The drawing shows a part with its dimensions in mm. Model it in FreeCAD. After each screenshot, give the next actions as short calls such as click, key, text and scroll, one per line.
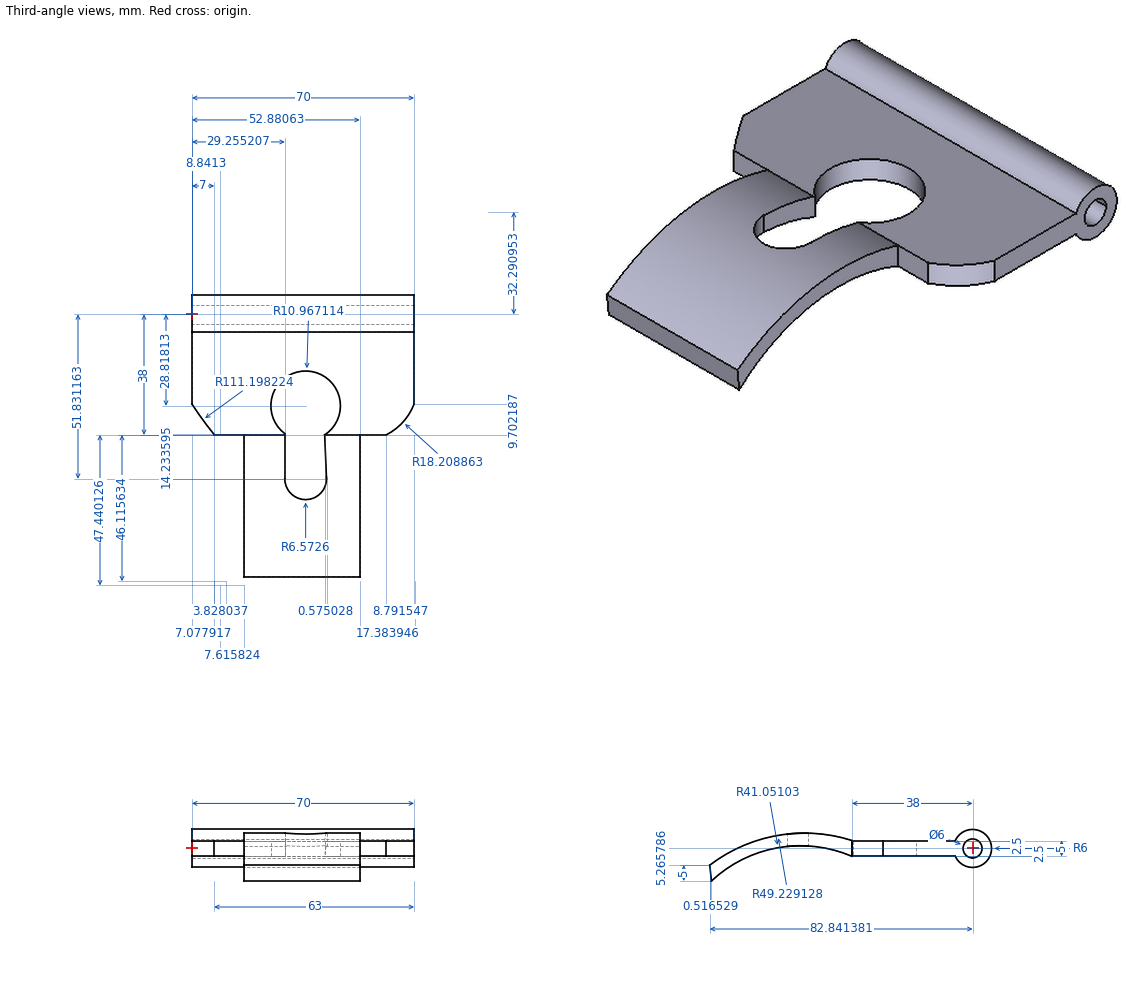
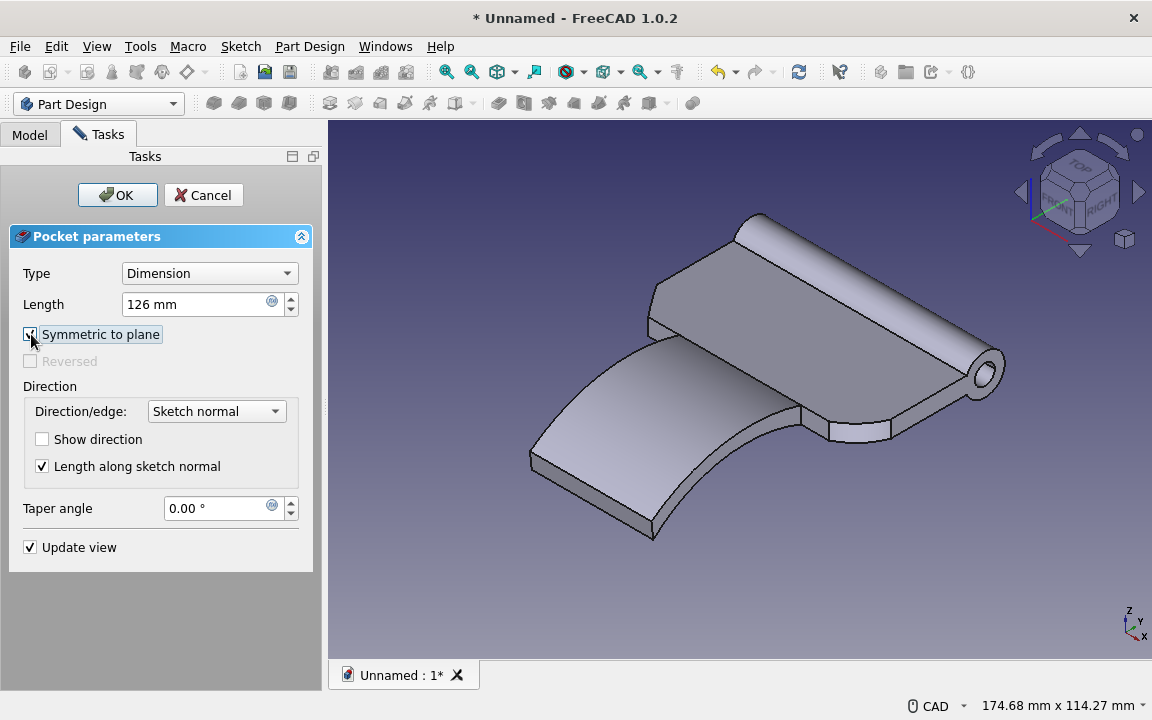
click(118, 195)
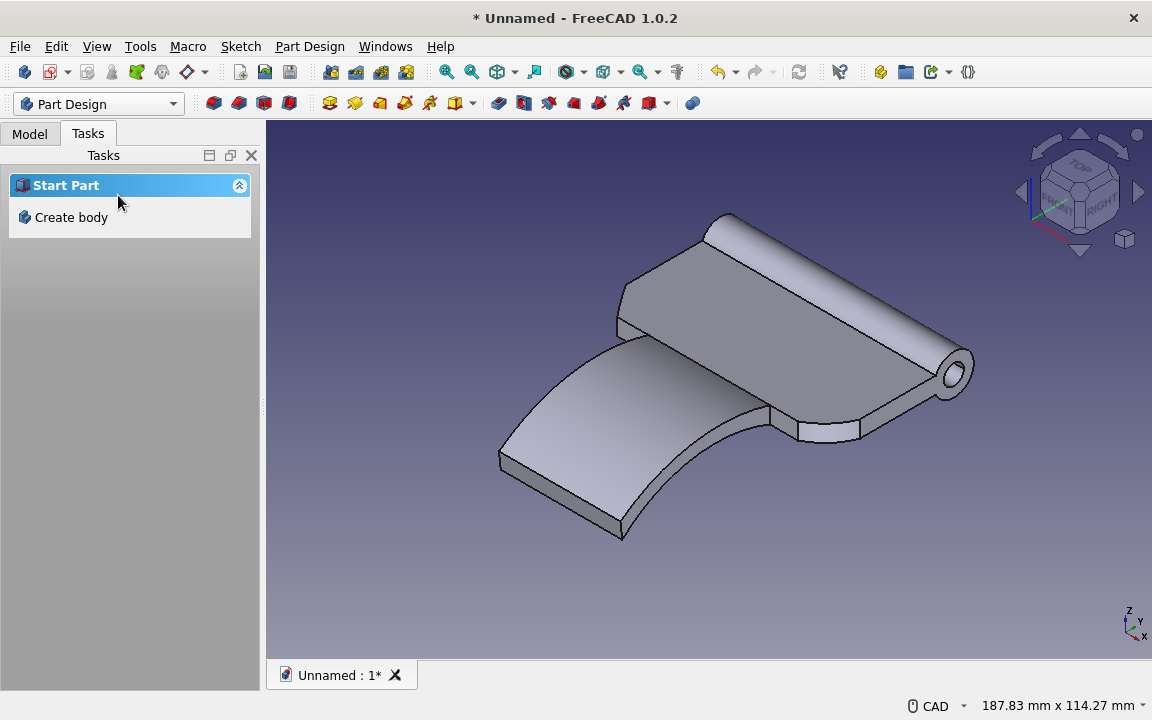
key(5)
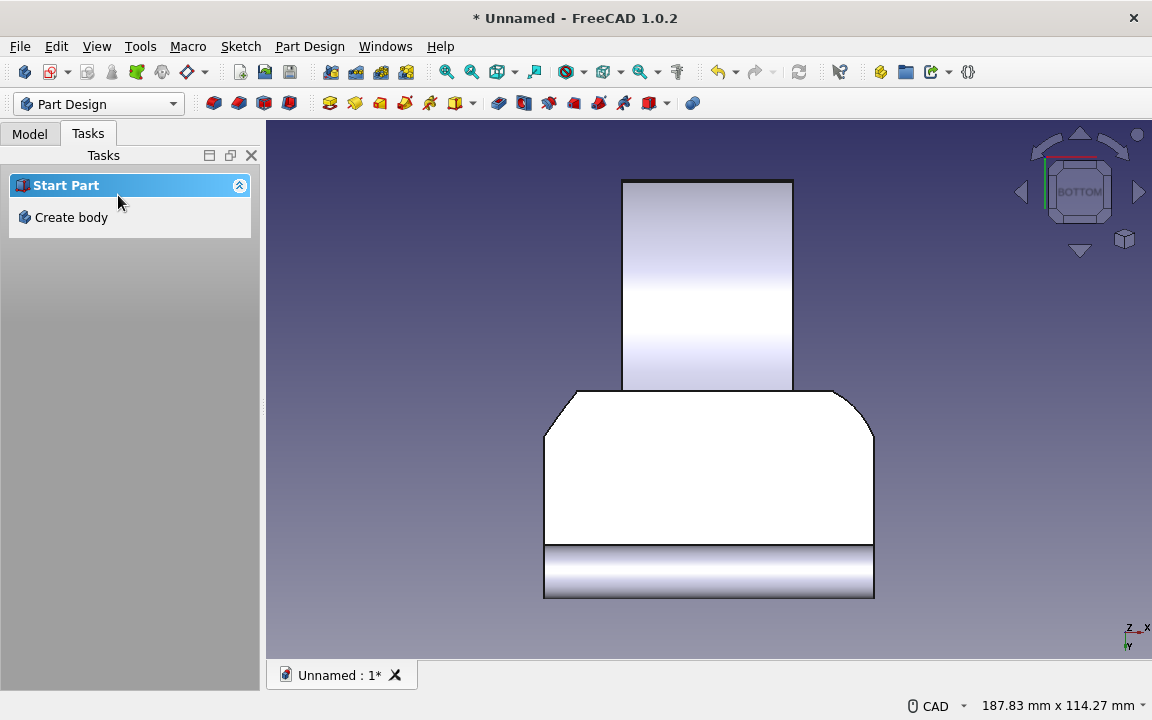
click(756, 467)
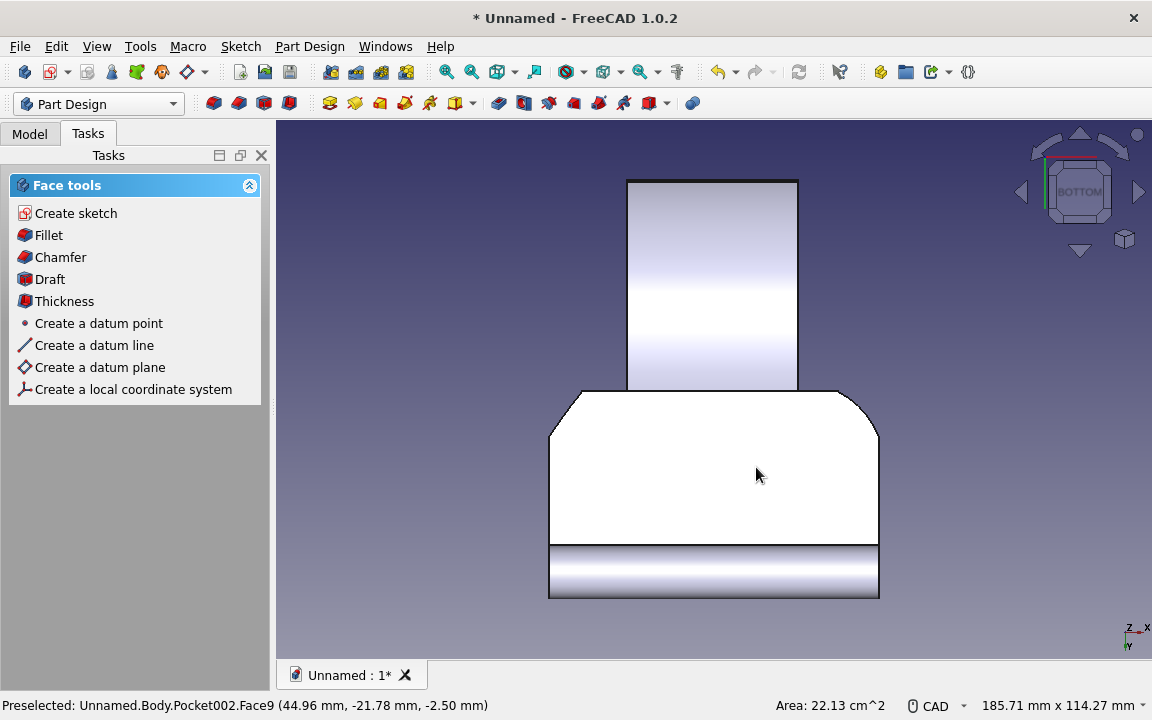
click(50, 72)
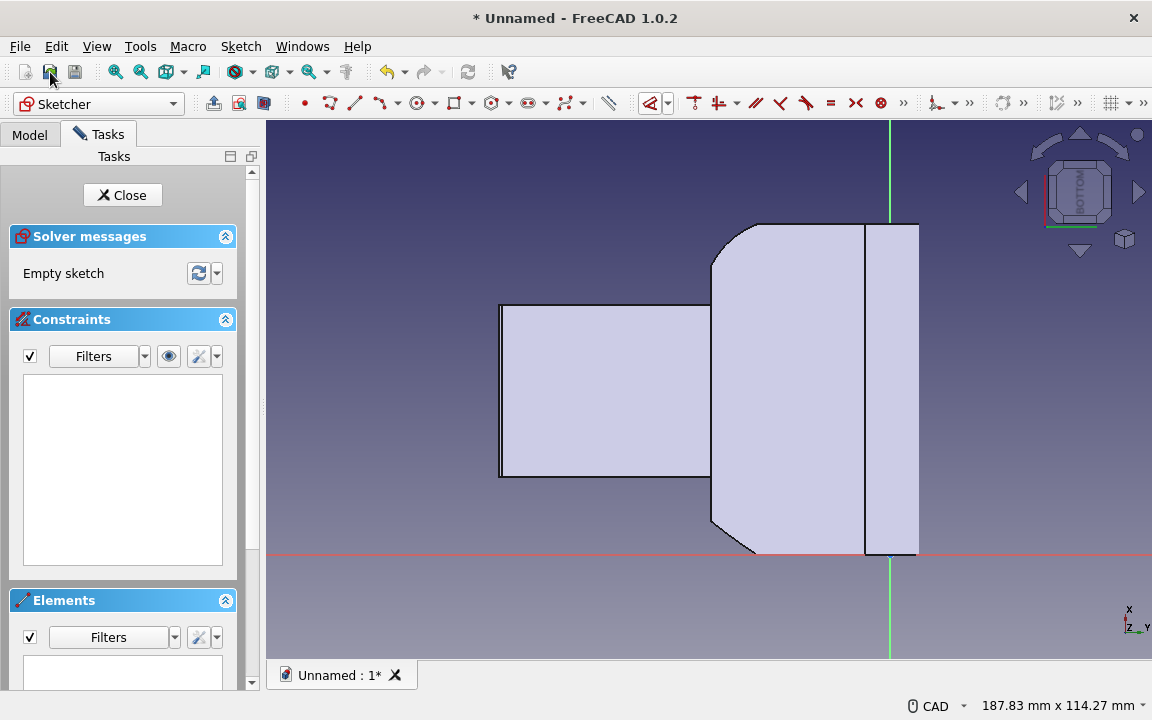
click(264, 104)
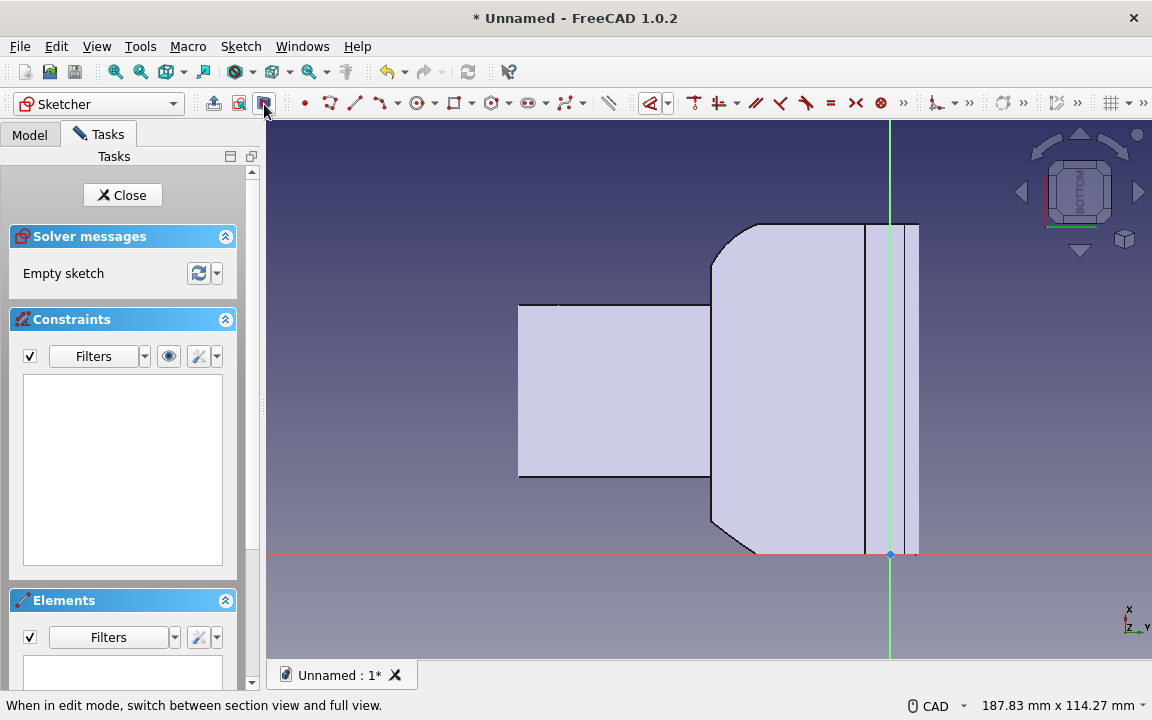
scroll(889, 534, up, 3)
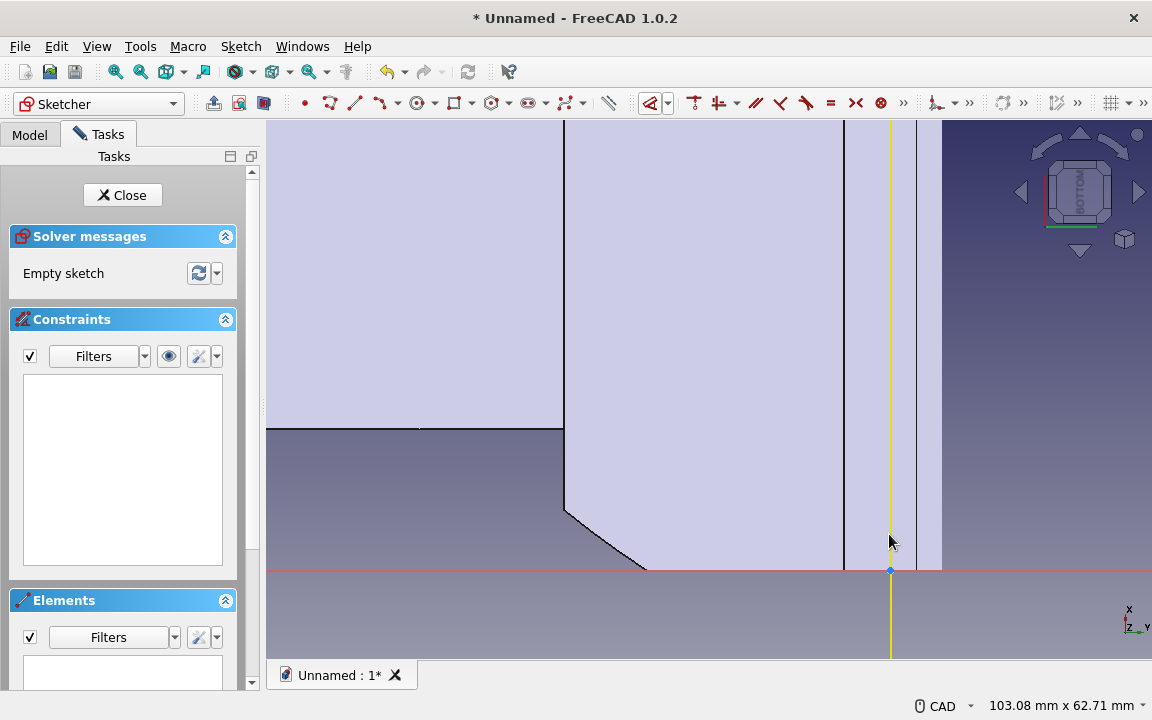
click(355, 104)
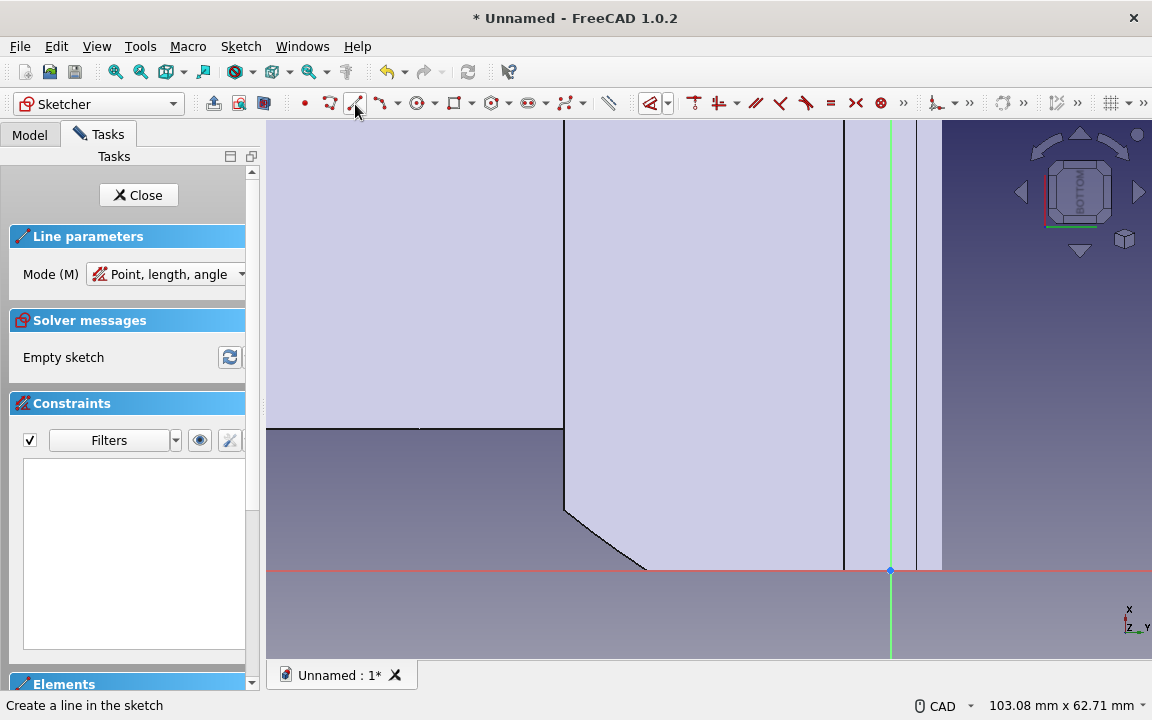
click(445, 319)
click(568, 319)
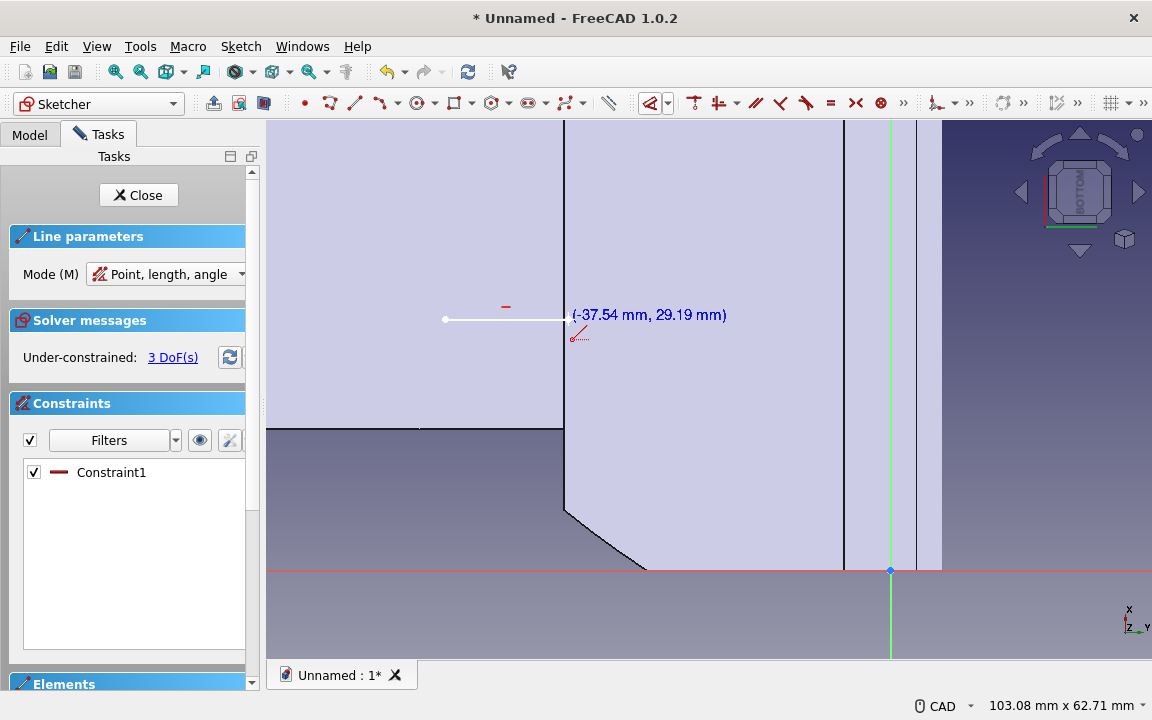
click(564, 211)
click(445, 204)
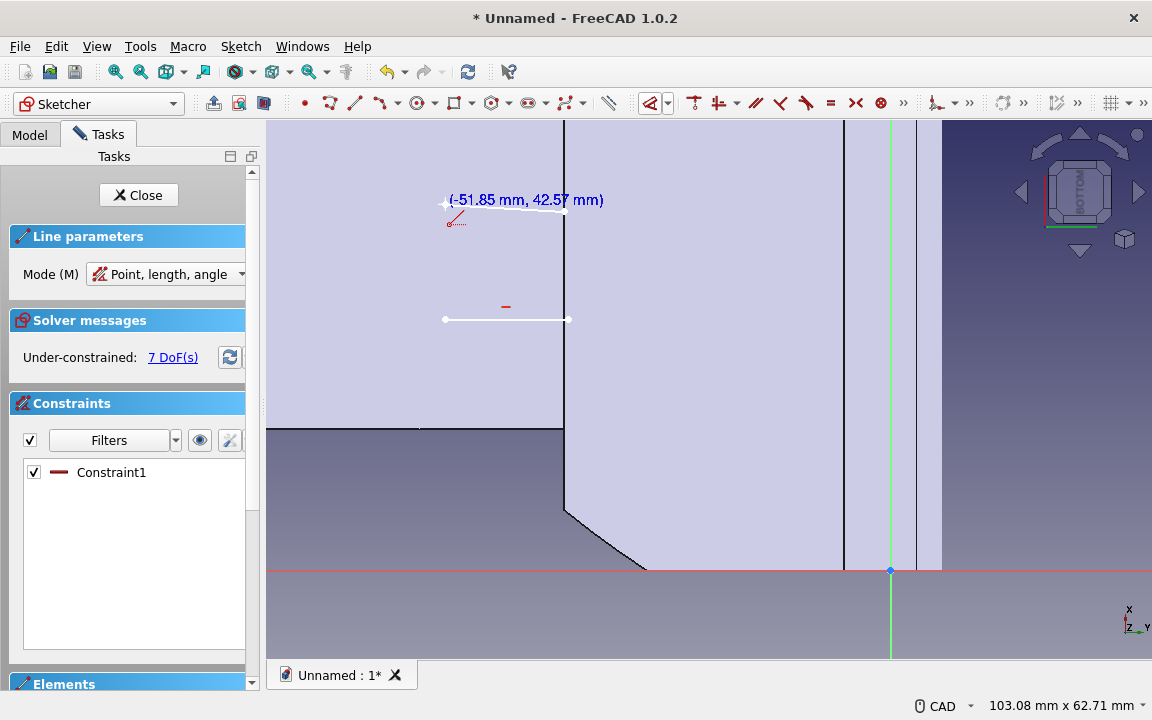
click(380, 104)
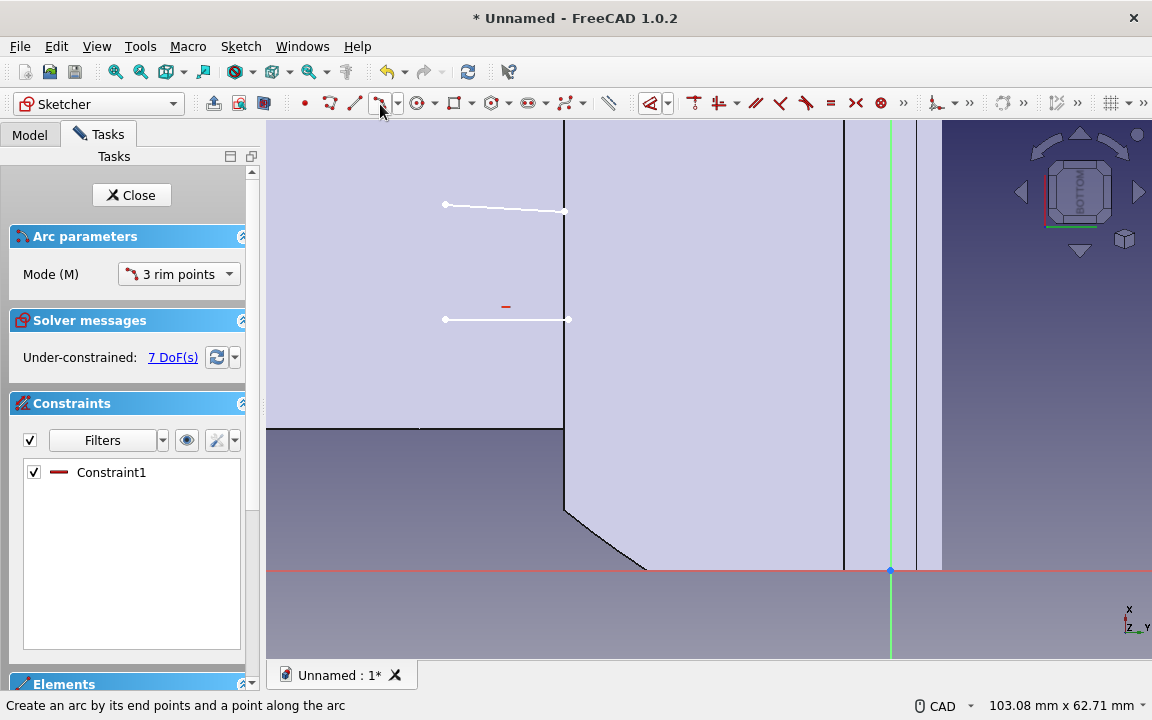
click(568, 320)
click(564, 212)
click(737, 260)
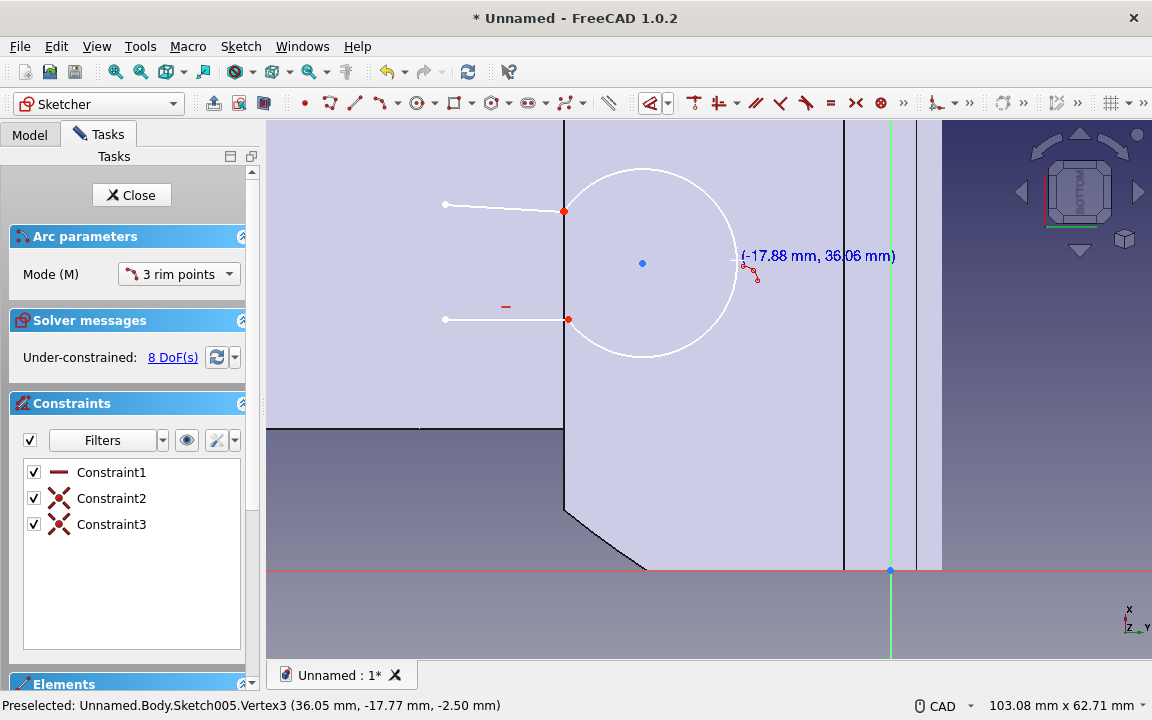
click(445, 205)
click(445, 320)
click(389, 263)
key(Escape)